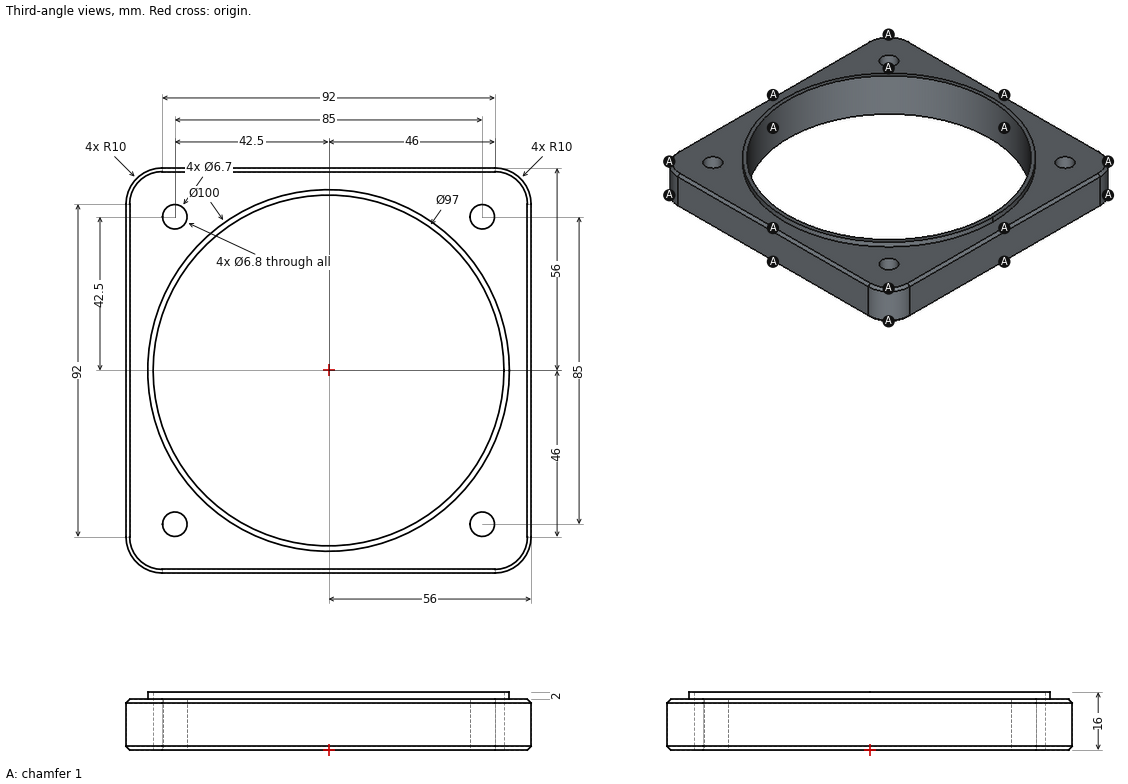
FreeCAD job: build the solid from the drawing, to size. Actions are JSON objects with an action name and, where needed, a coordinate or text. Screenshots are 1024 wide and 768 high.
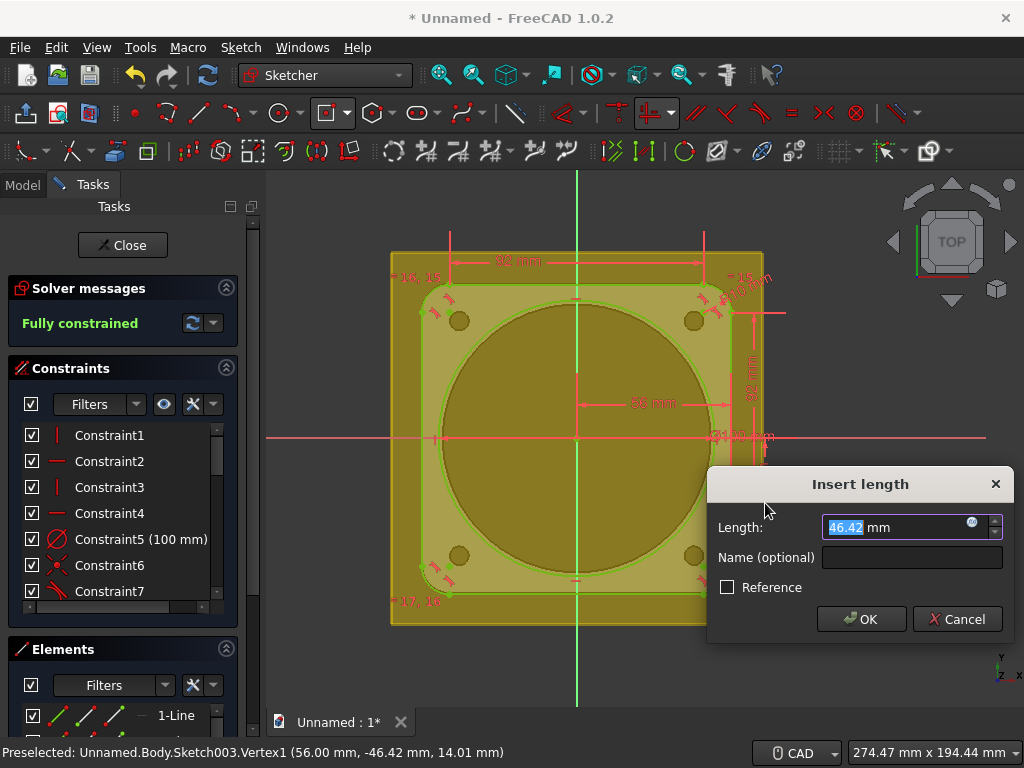
{"action": "type", "text": "46"}
{"action": "key", "text": "Return"}
{"action": "key", "text": "Escape"}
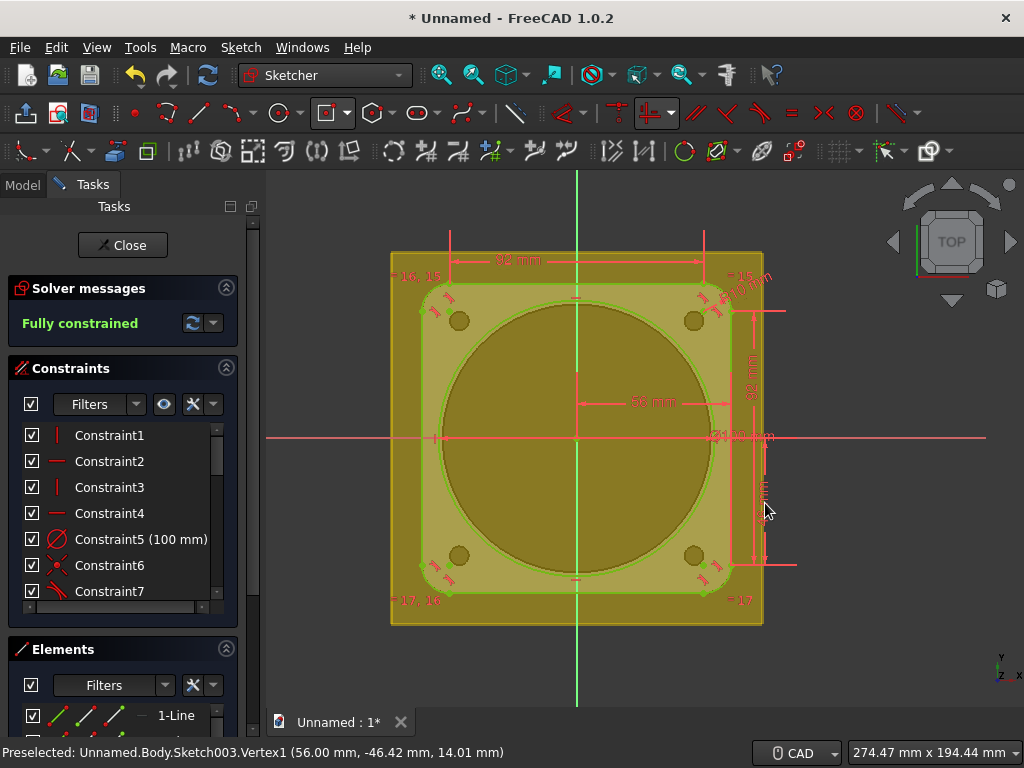
{"action": "left_click", "coordinate": [123, 245]}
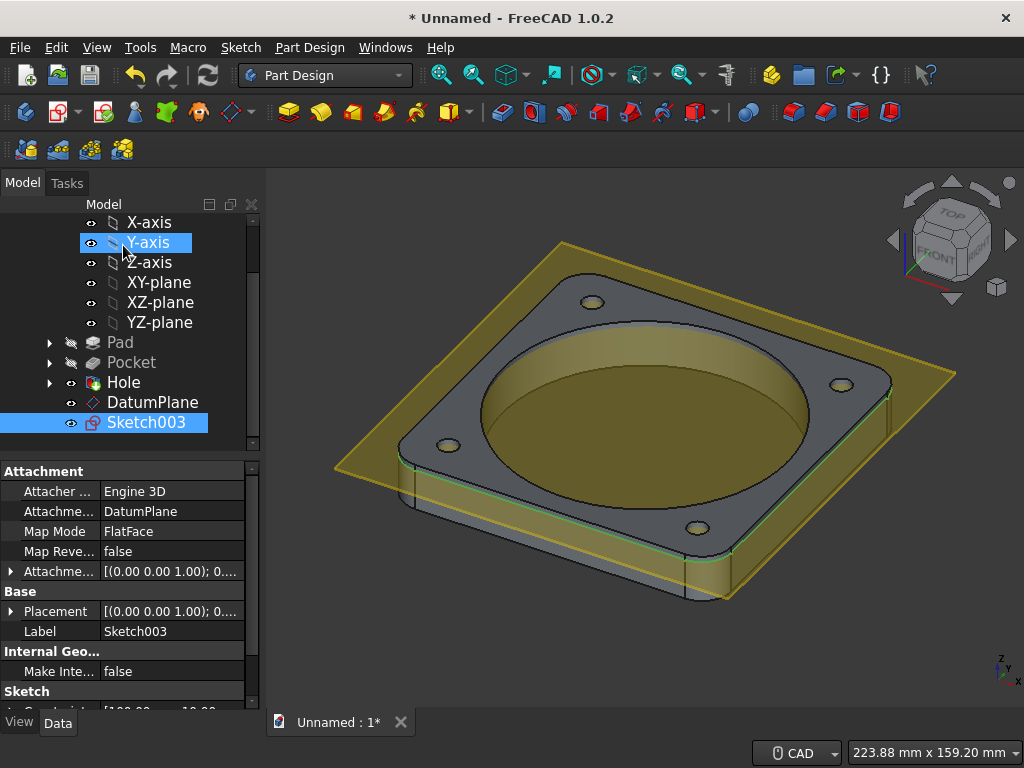
{"action": "left_click", "coordinate": [504, 112]}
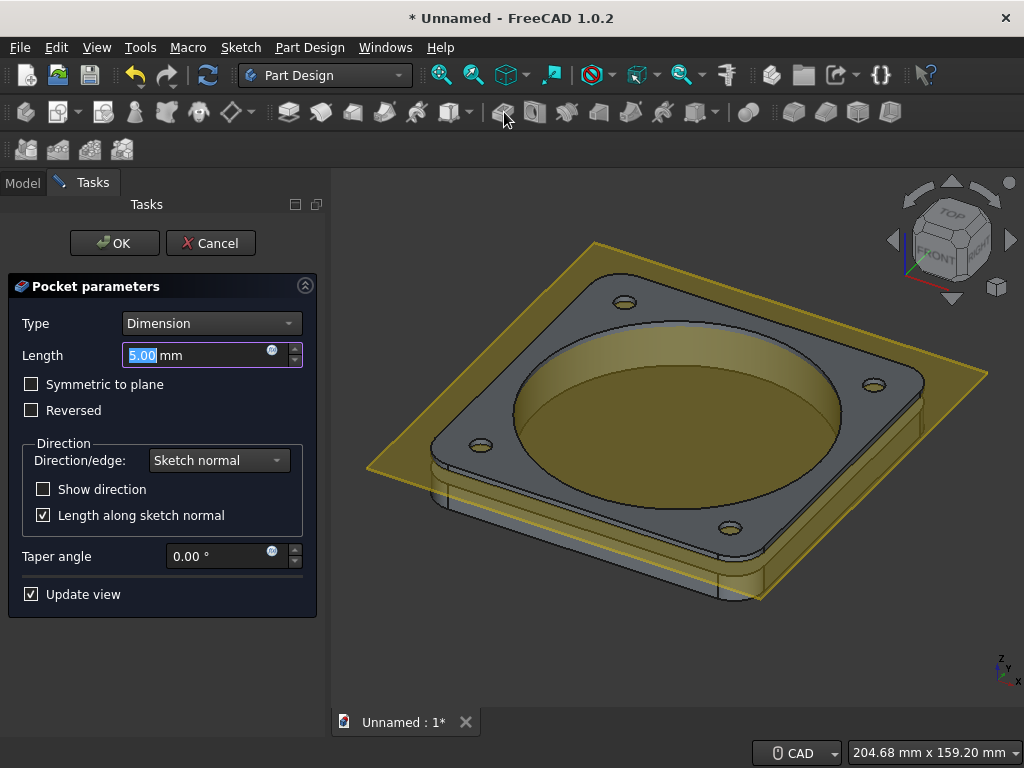
{"action": "type", "text": "2"}
{"action": "key", "text": "Tab"}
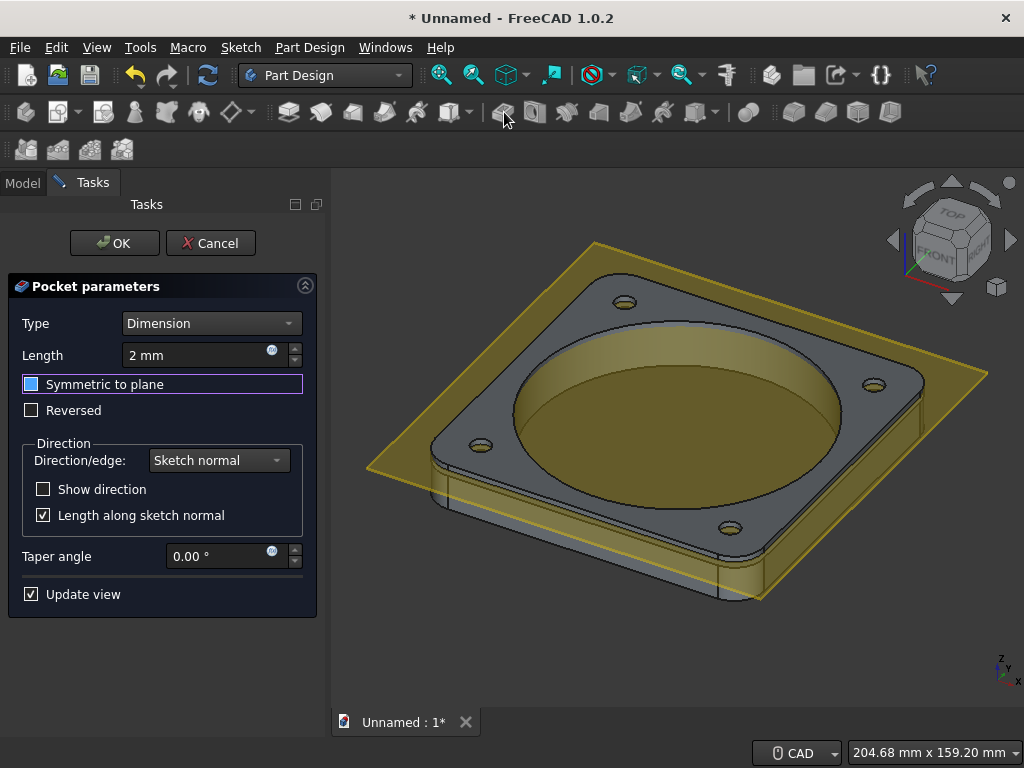
{"action": "left_click", "coordinate": [30, 410]}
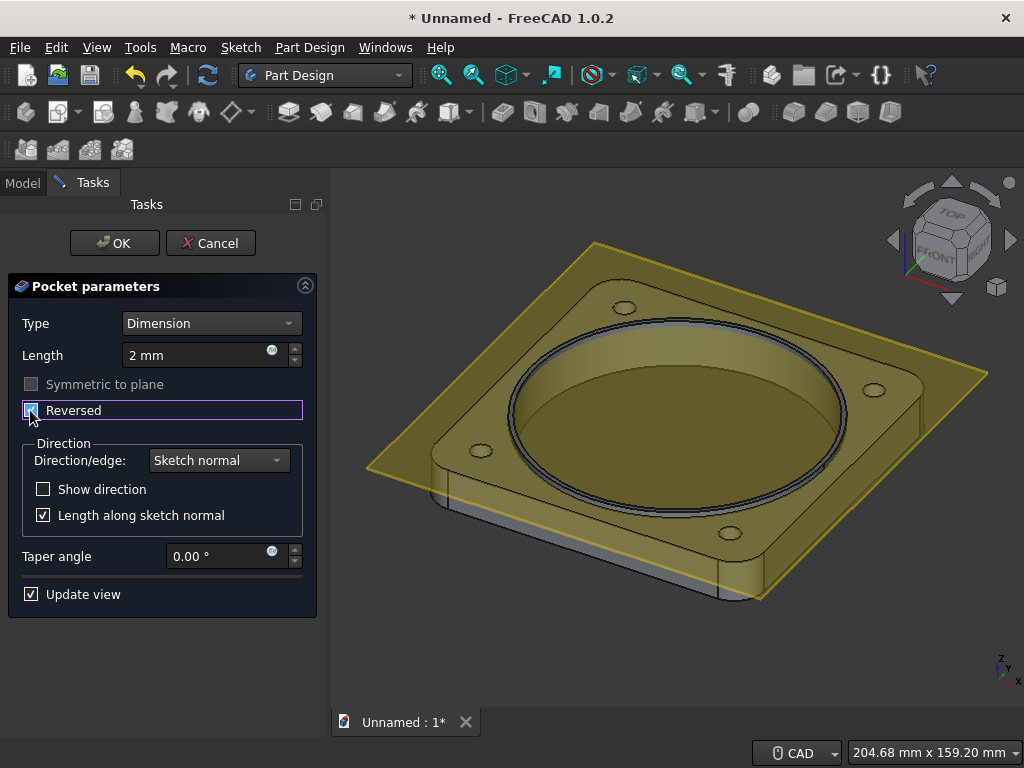
{"action": "left_click", "coordinate": [115, 243]}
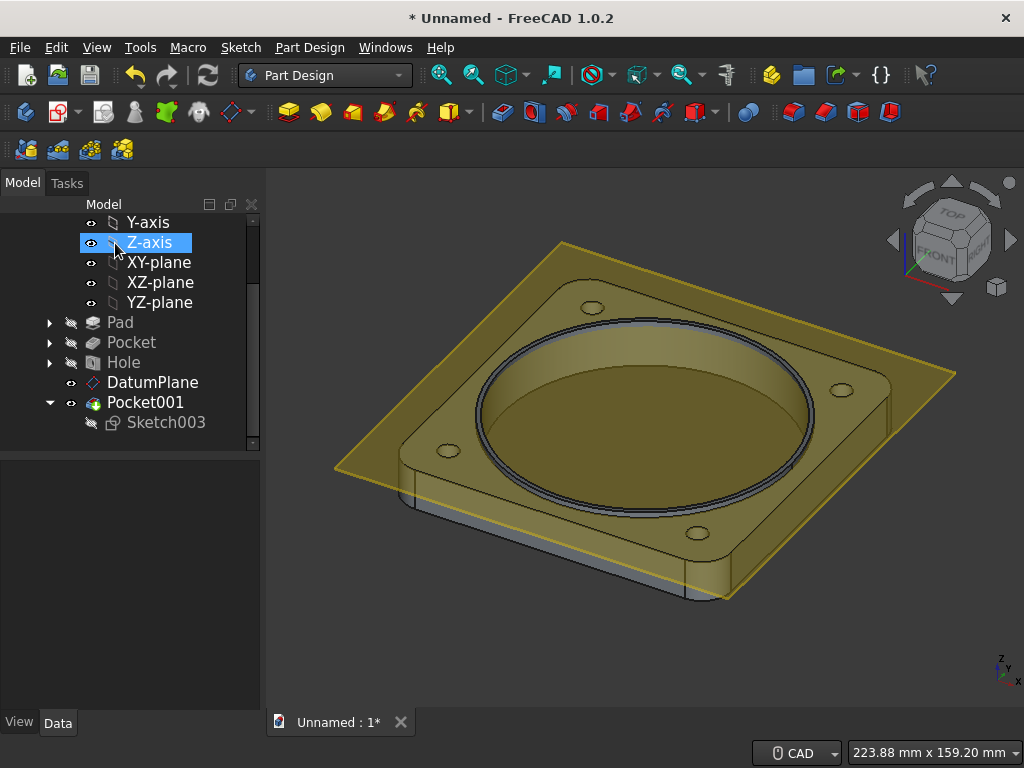
{"action": "left_click", "coordinate": [116, 383]}
{"action": "key", "text": "space"}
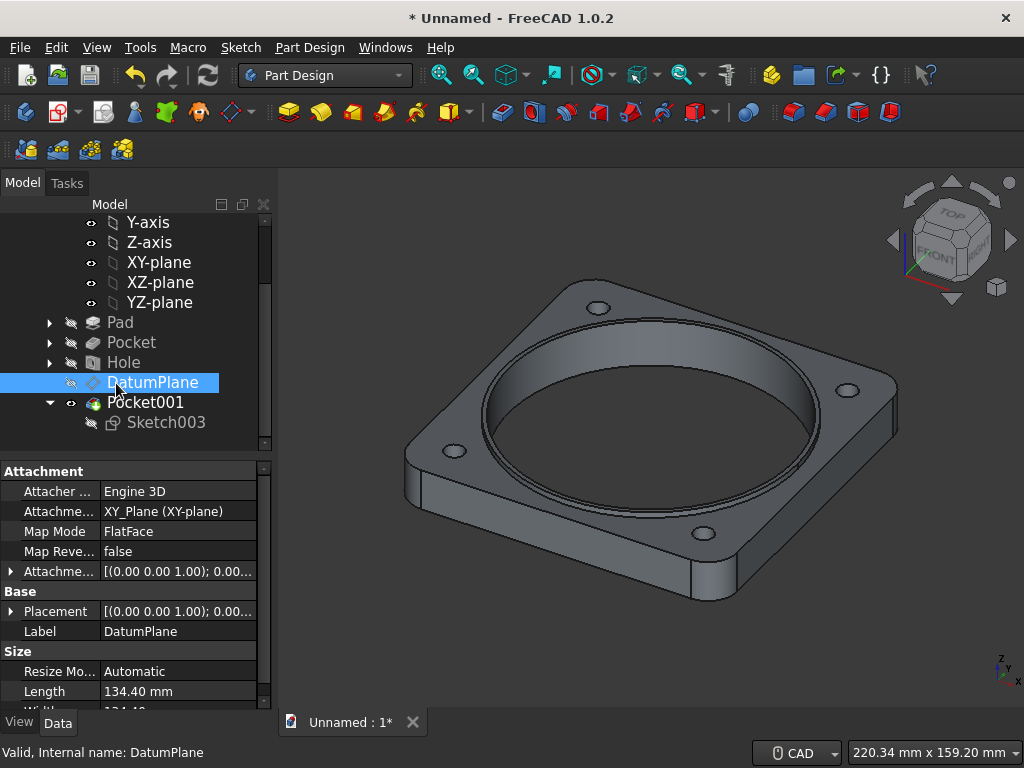
{"action": "left_click", "coordinate": [895, 379]}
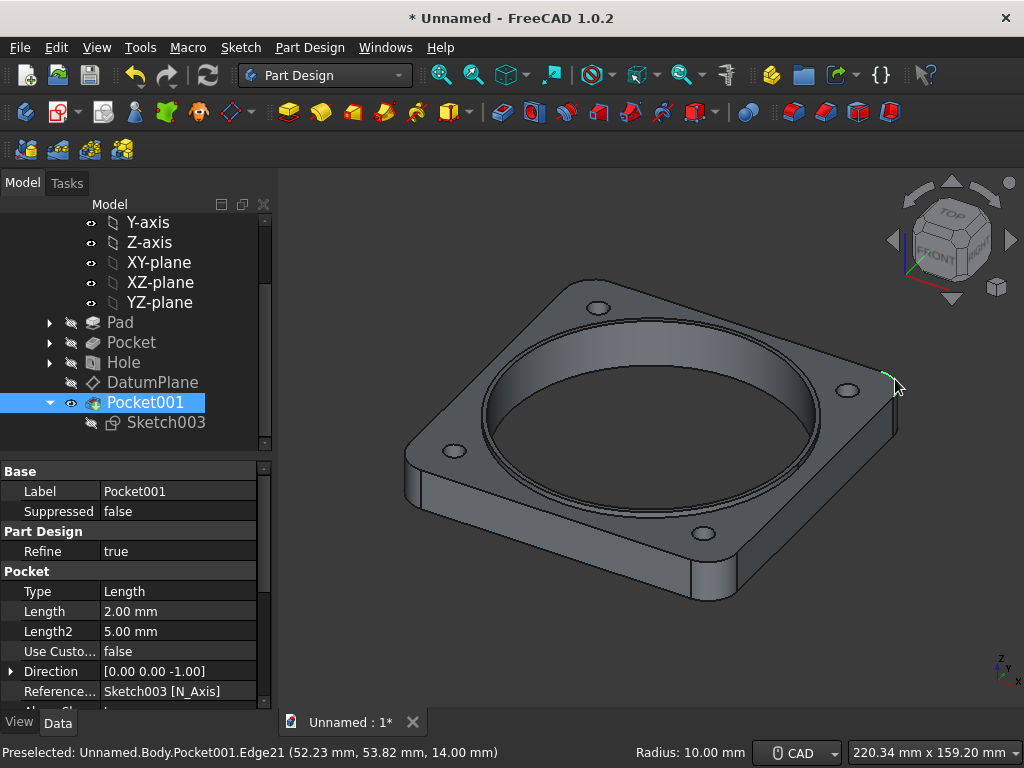
{"action": "left_click", "coordinate": [815, 474], "text": "ctrl"}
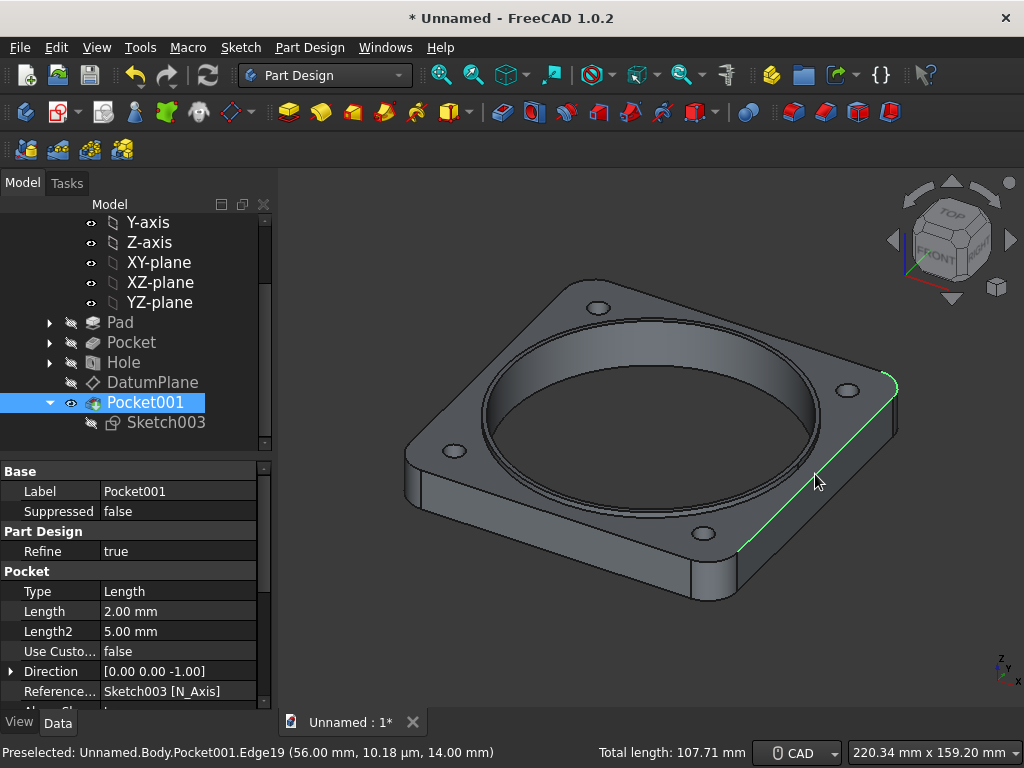
{"action": "left_click", "coordinate": [717, 561], "text": "ctrl"}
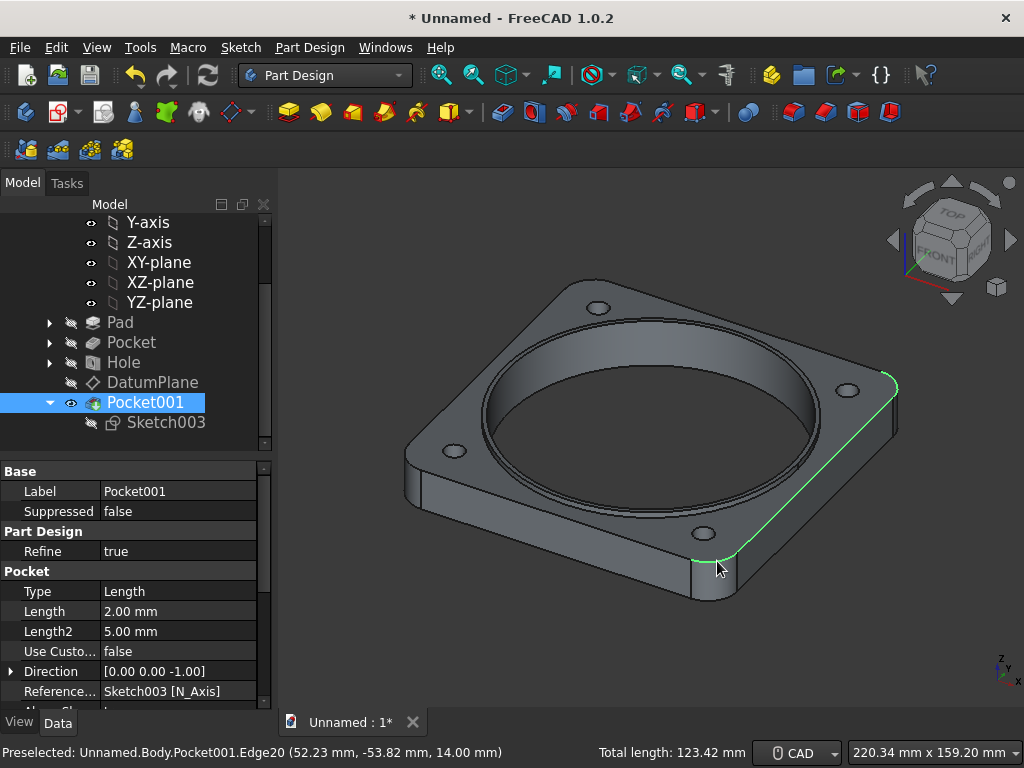
{"action": "left_click", "coordinate": [556, 514], "text": "ctrl"}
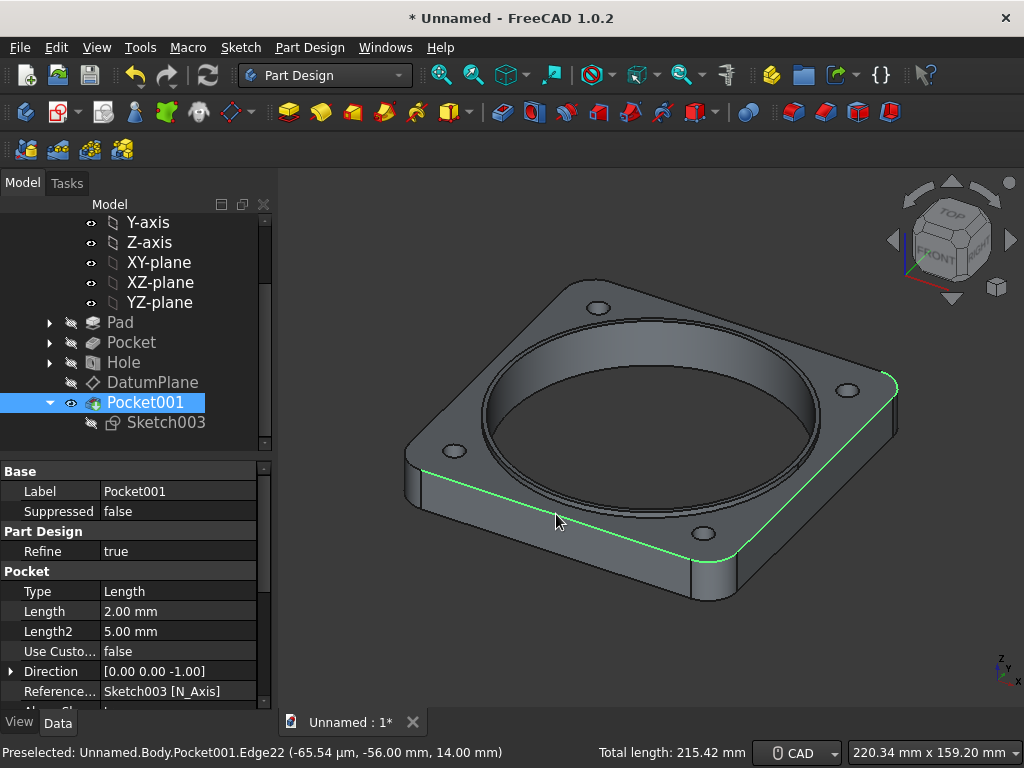
{"action": "left_click", "coordinate": [406, 458], "text": "ctrl"}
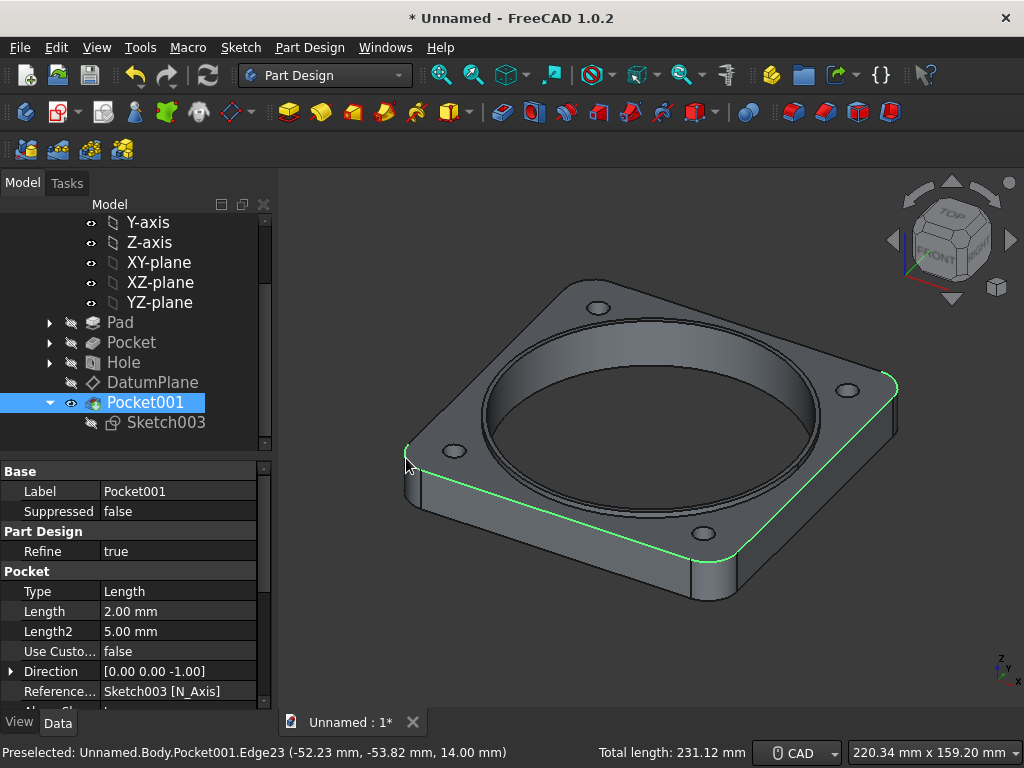
{"action": "left_click", "coordinate": [571, 283], "text": "ctrl"}